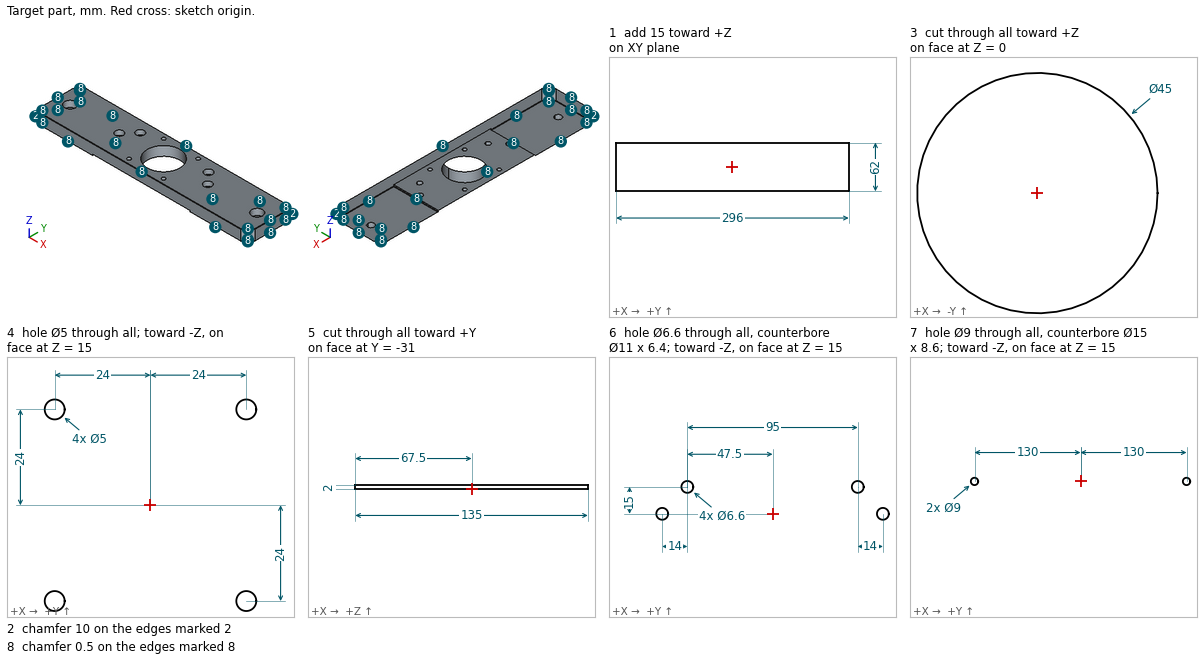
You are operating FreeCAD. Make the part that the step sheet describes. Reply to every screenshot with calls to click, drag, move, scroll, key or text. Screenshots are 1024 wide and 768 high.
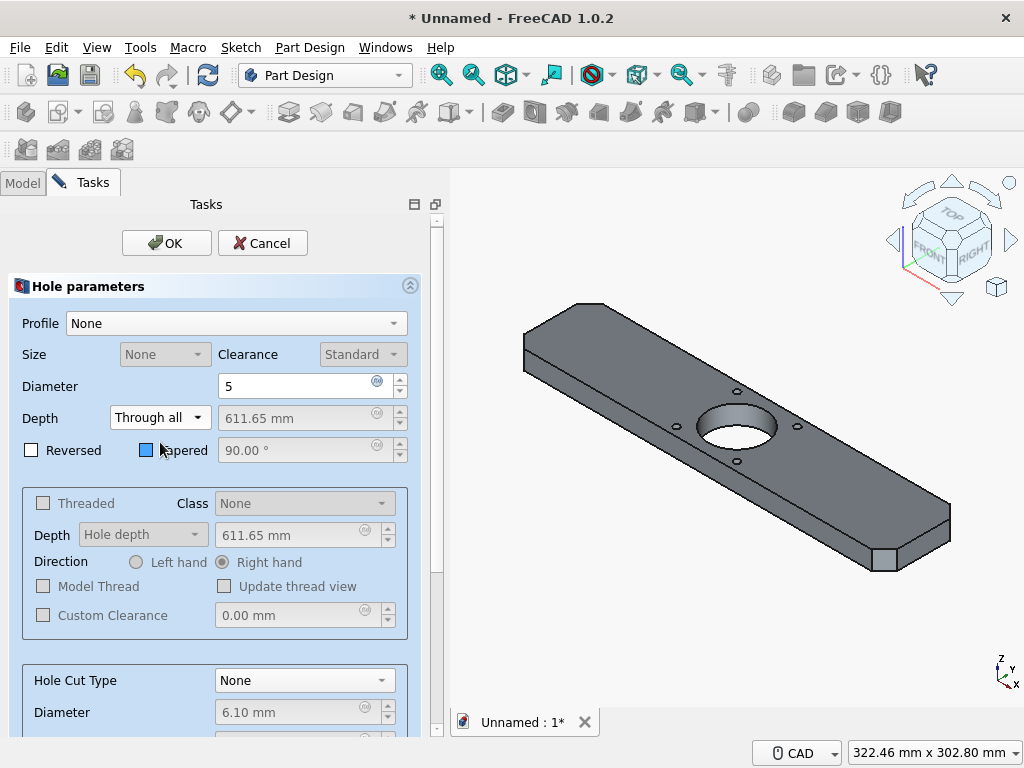
click(167, 243)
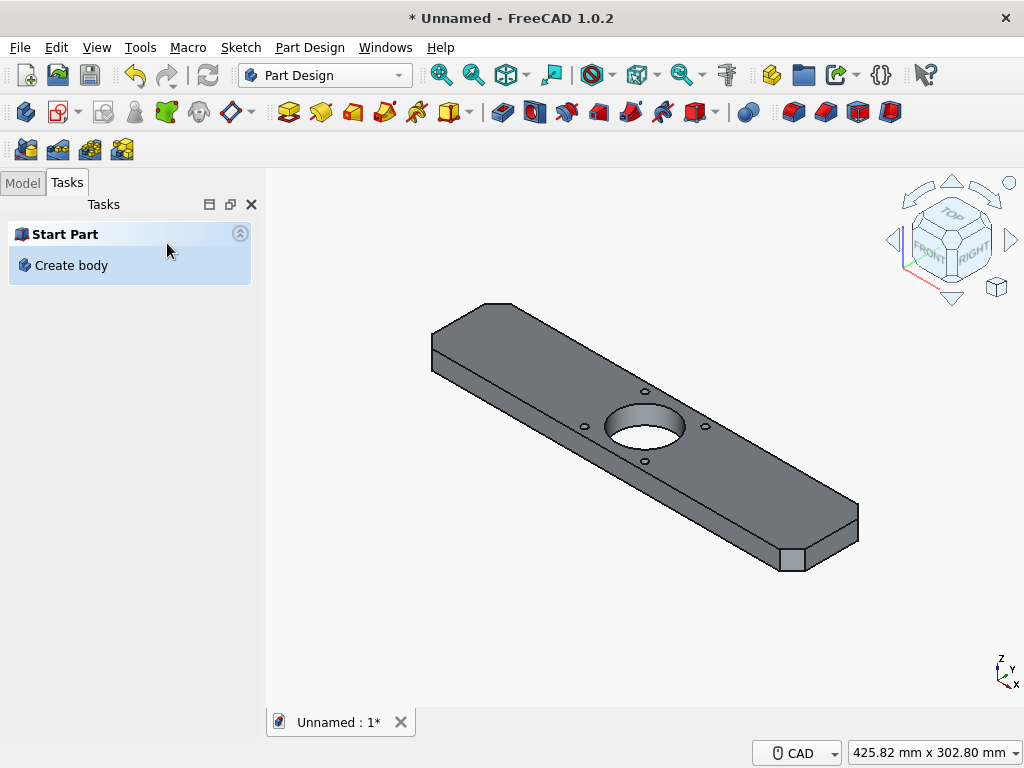
click(755, 545)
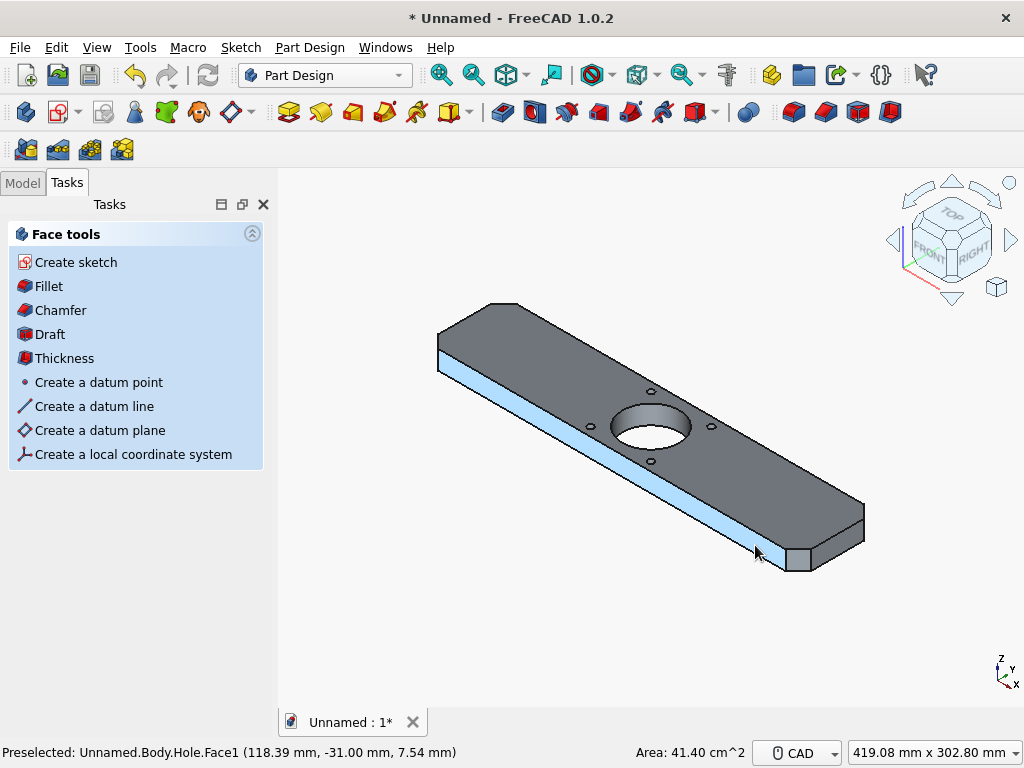
click(58, 112)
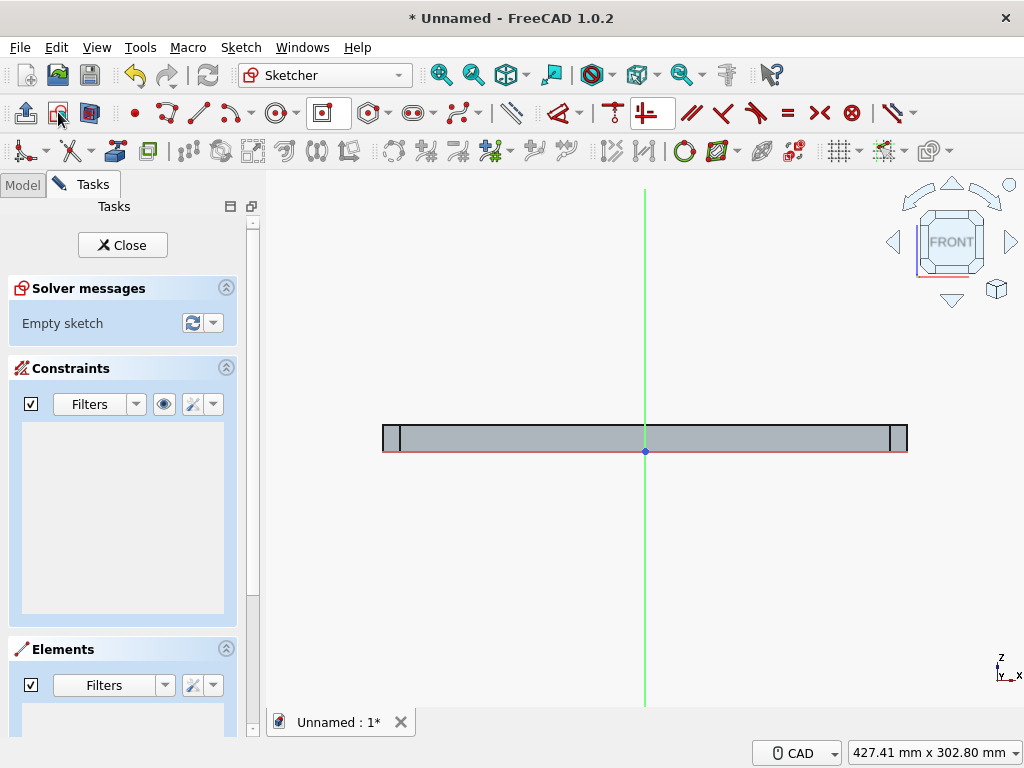
scroll(728, 464, up, 3)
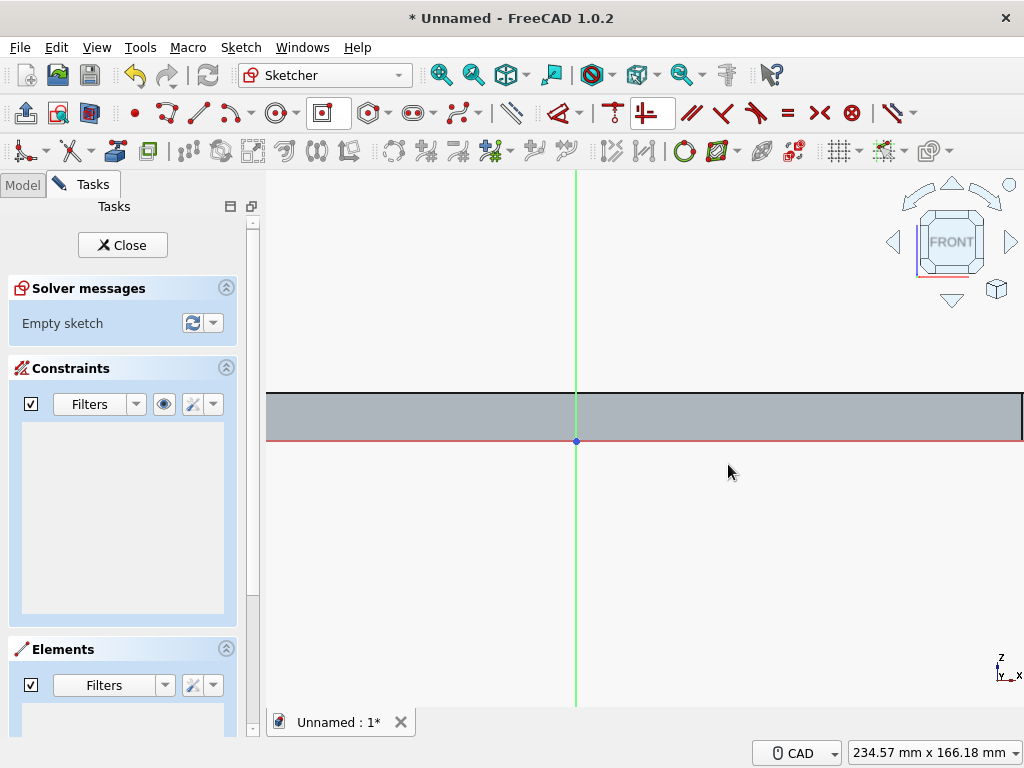
key(g)
key(r)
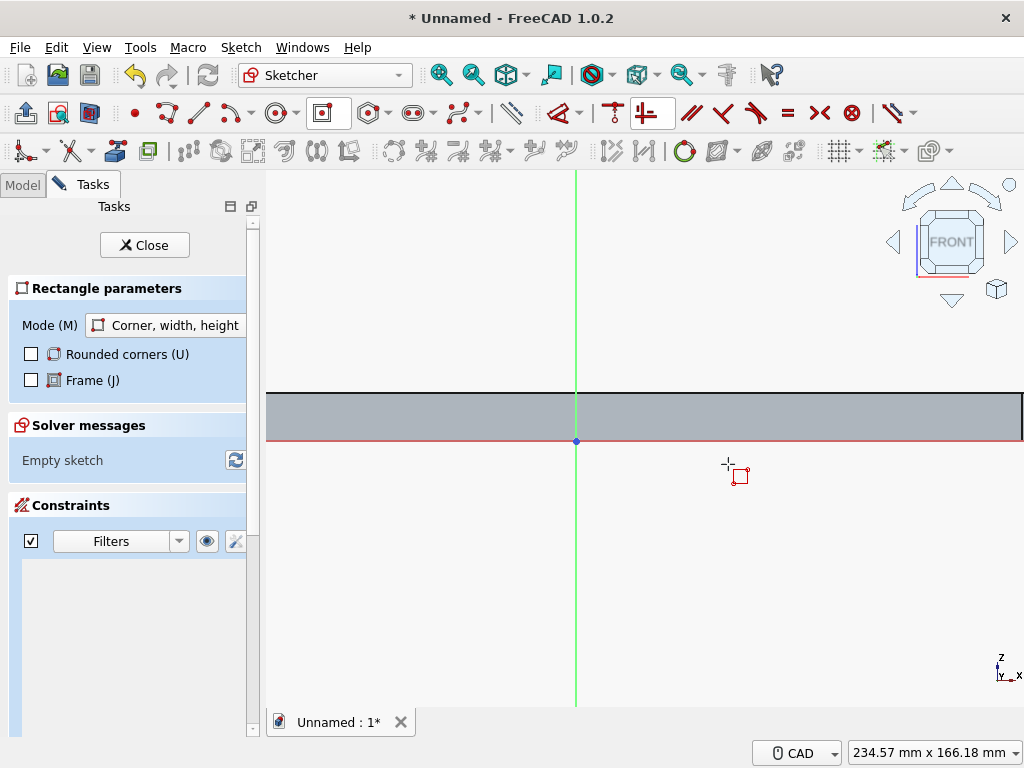
scroll(358, 435, up, 5)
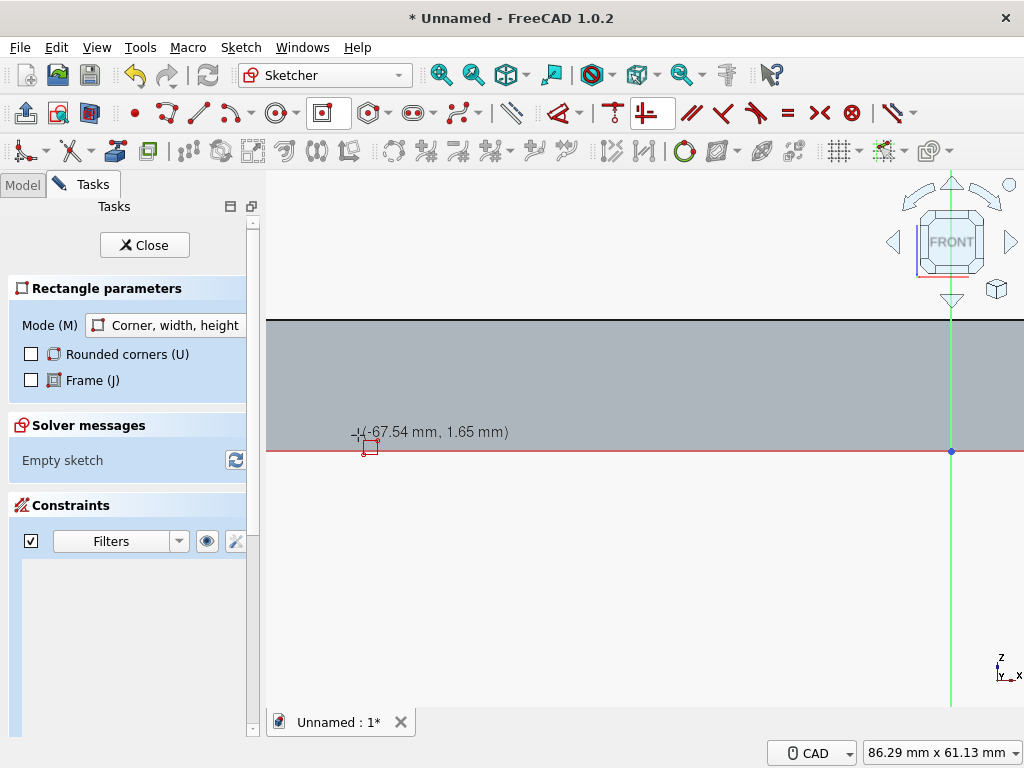
click(358, 434)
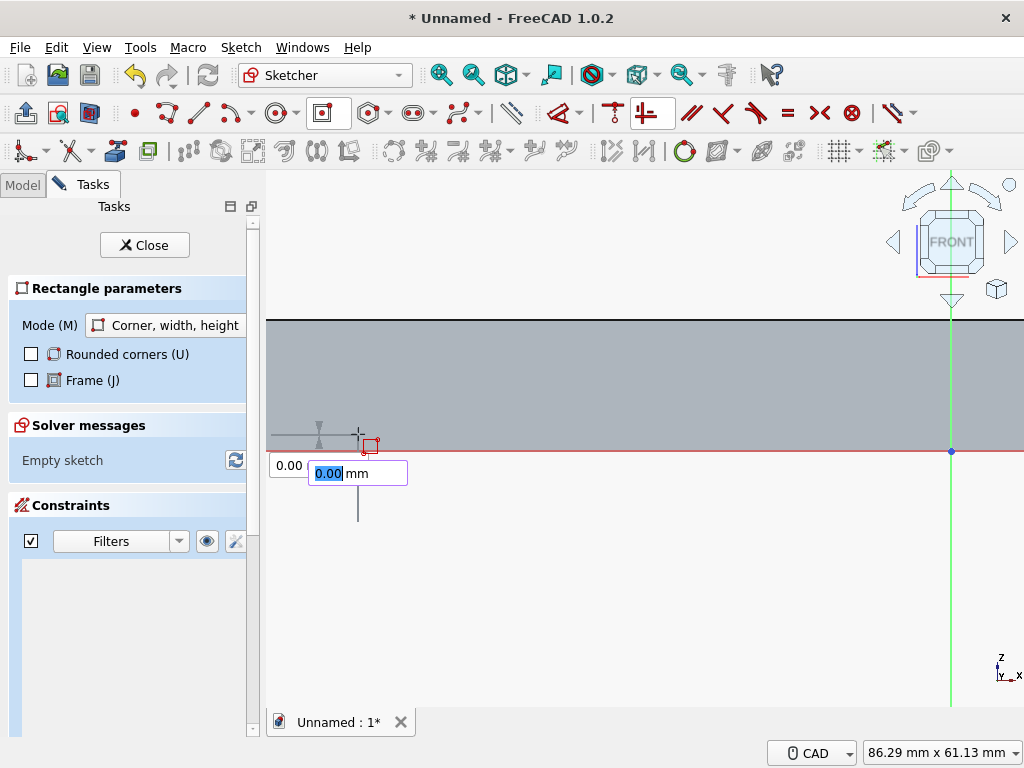
scroll(358, 436, down, 5)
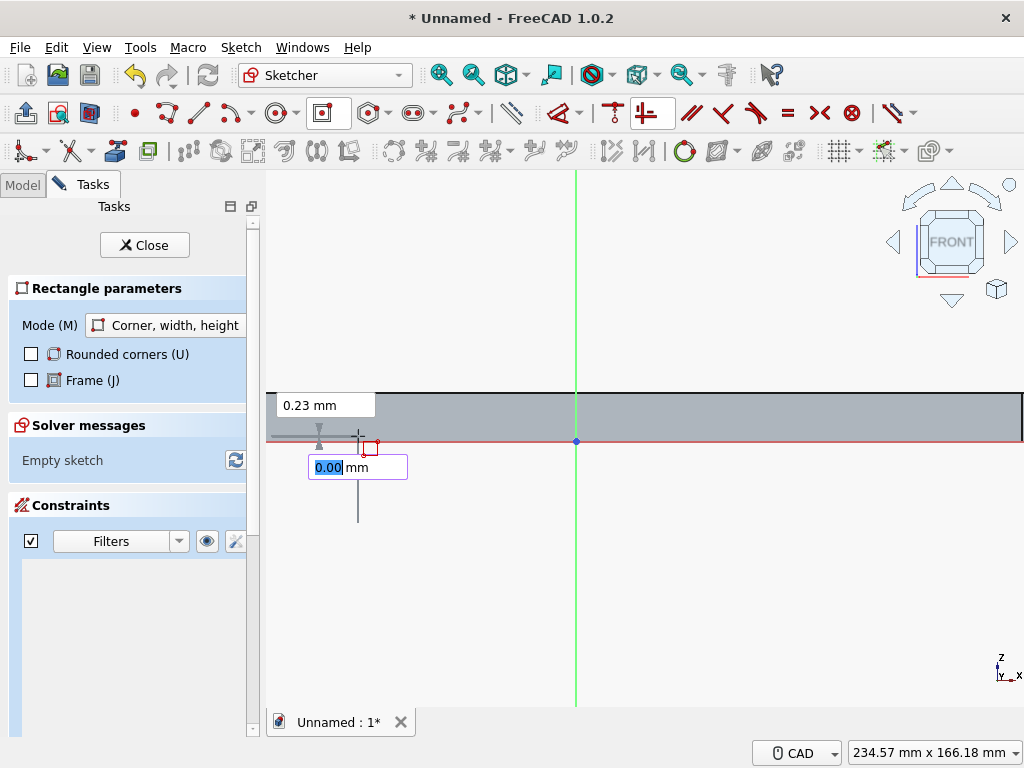
click(794, 442)
key(Escape)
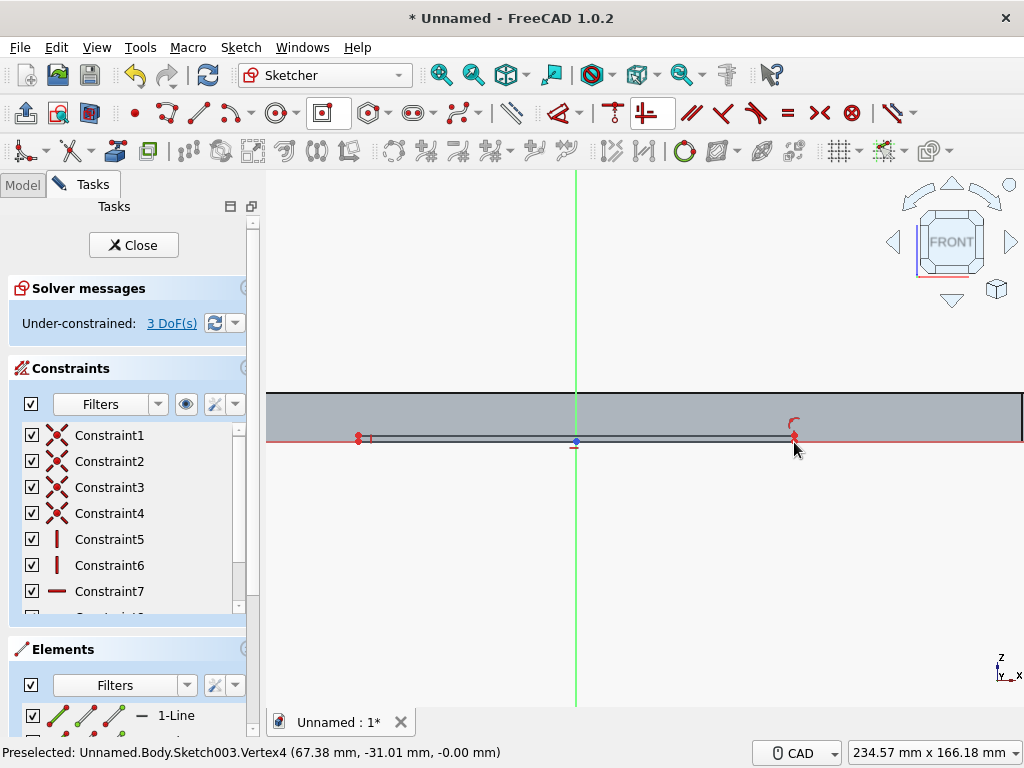
click(558, 114)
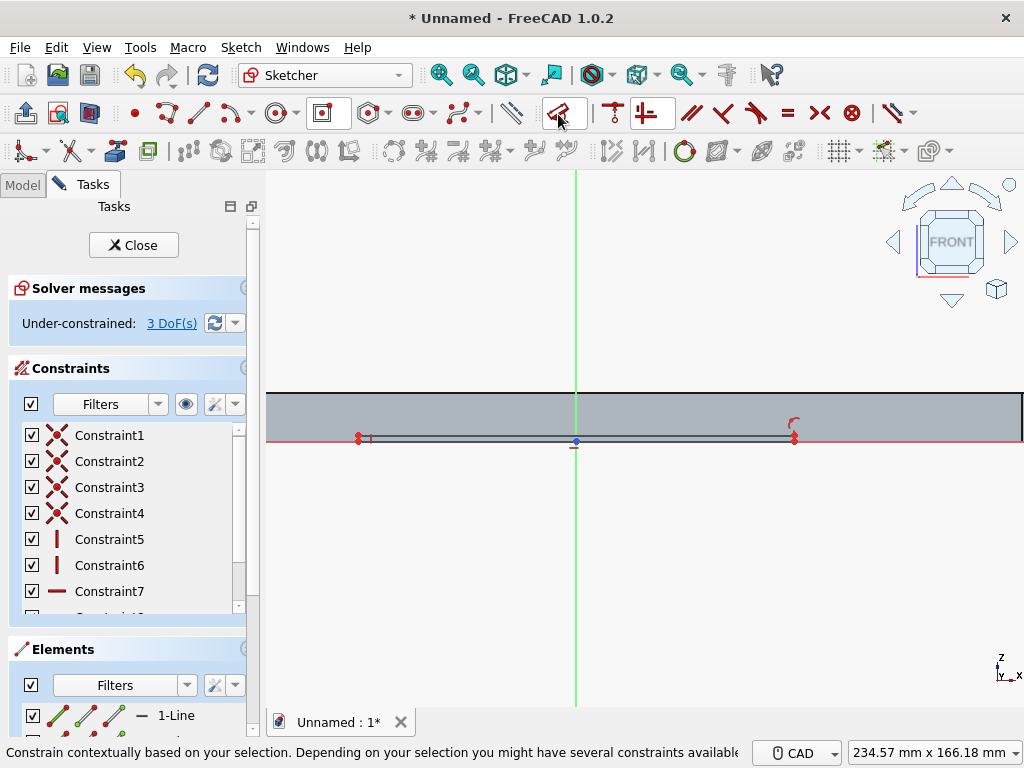
scroll(358, 439, up, 10)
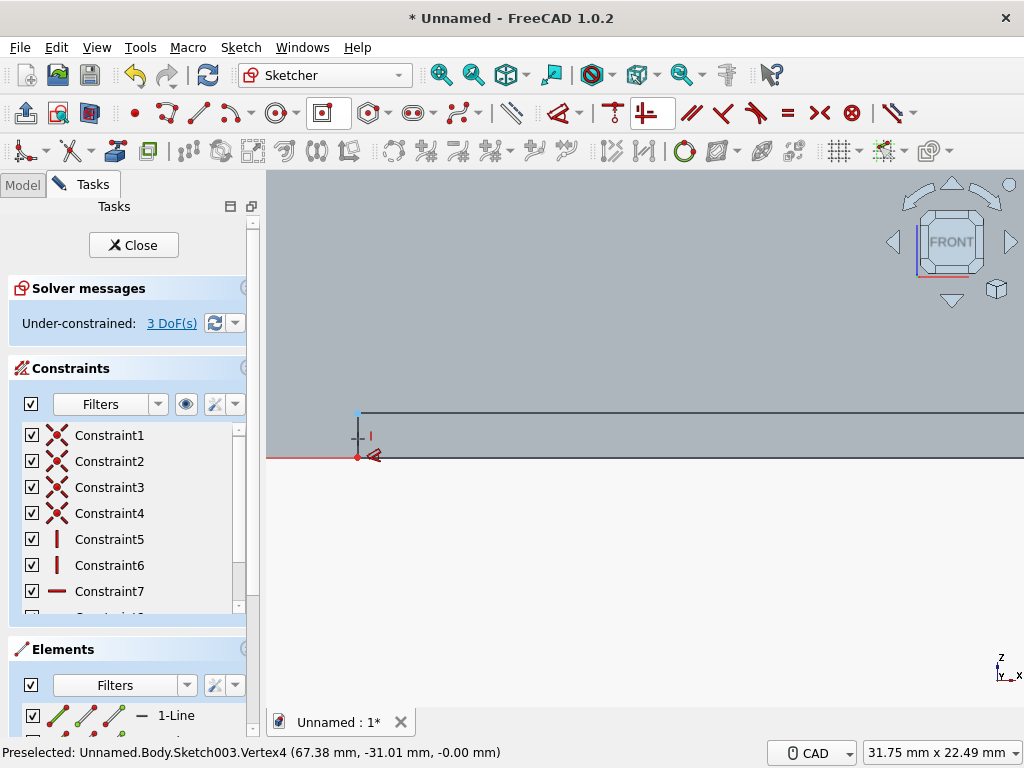
click(358, 435)
click(324, 435)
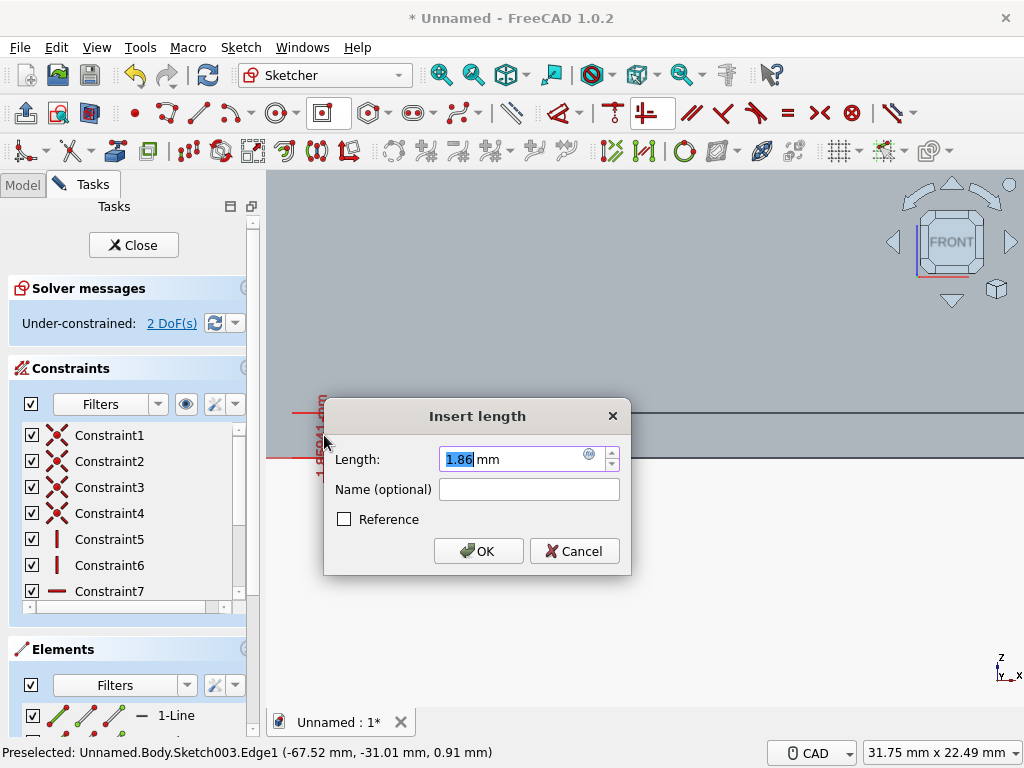
text(2)
key(Return)